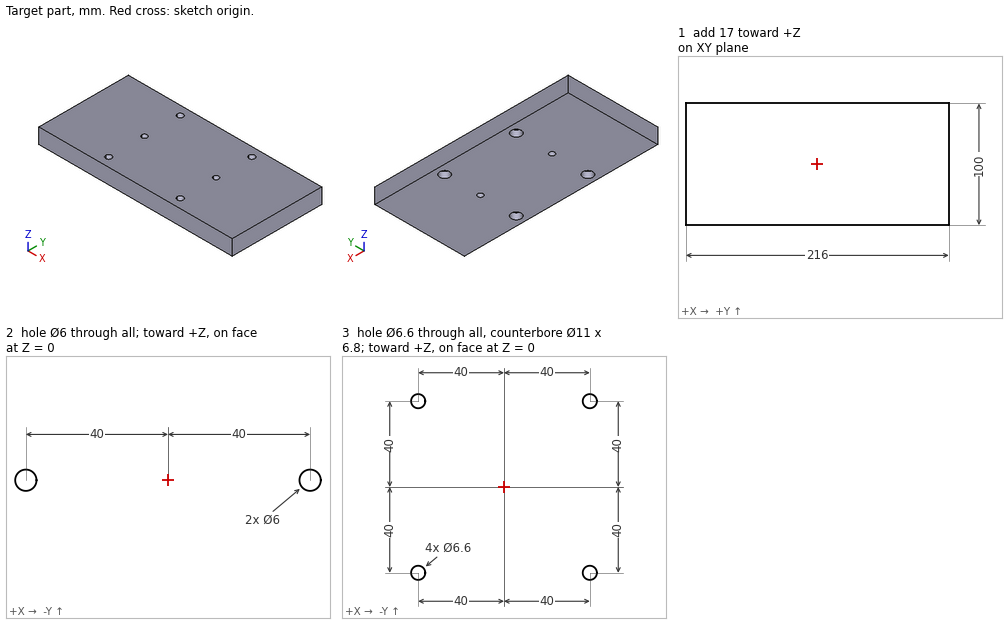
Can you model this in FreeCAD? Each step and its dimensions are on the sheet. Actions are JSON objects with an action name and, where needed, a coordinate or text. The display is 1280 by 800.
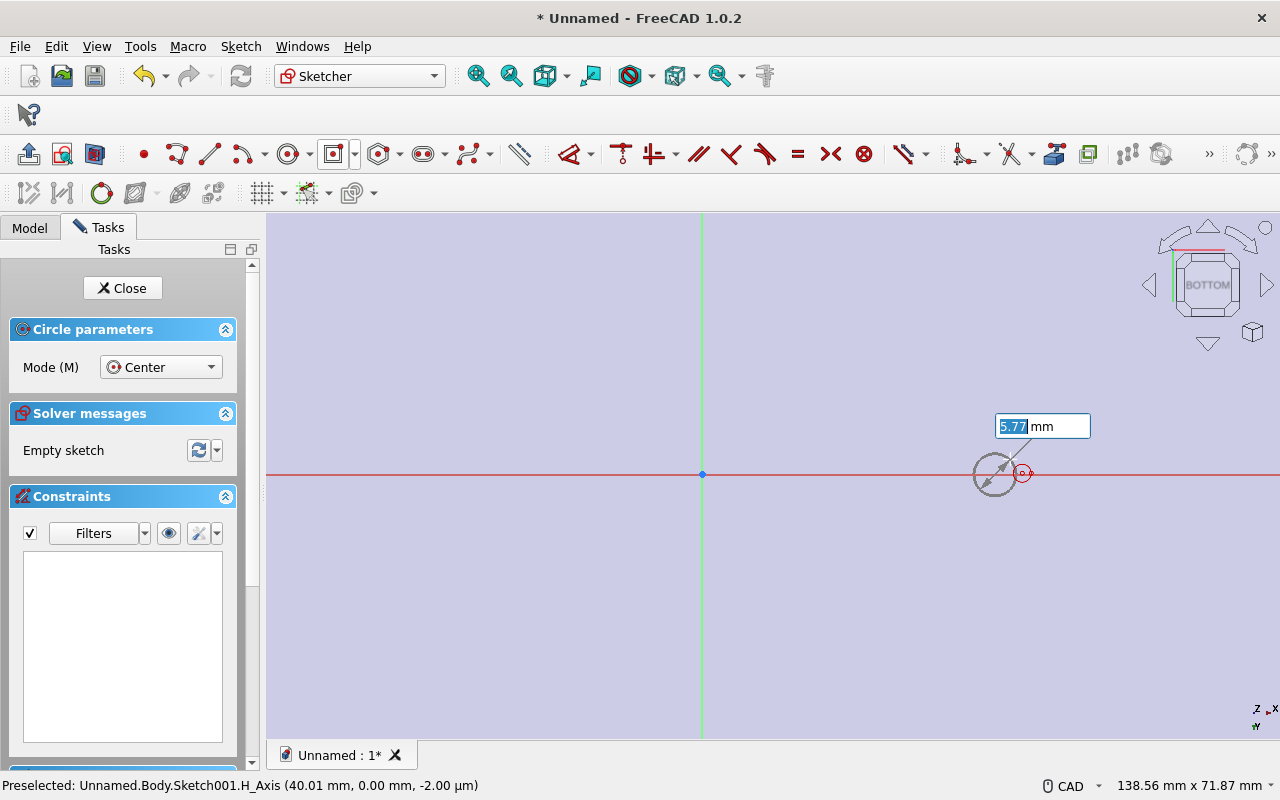
{"action": "type", "text": "6"}
{"action": "key", "text": "Return"}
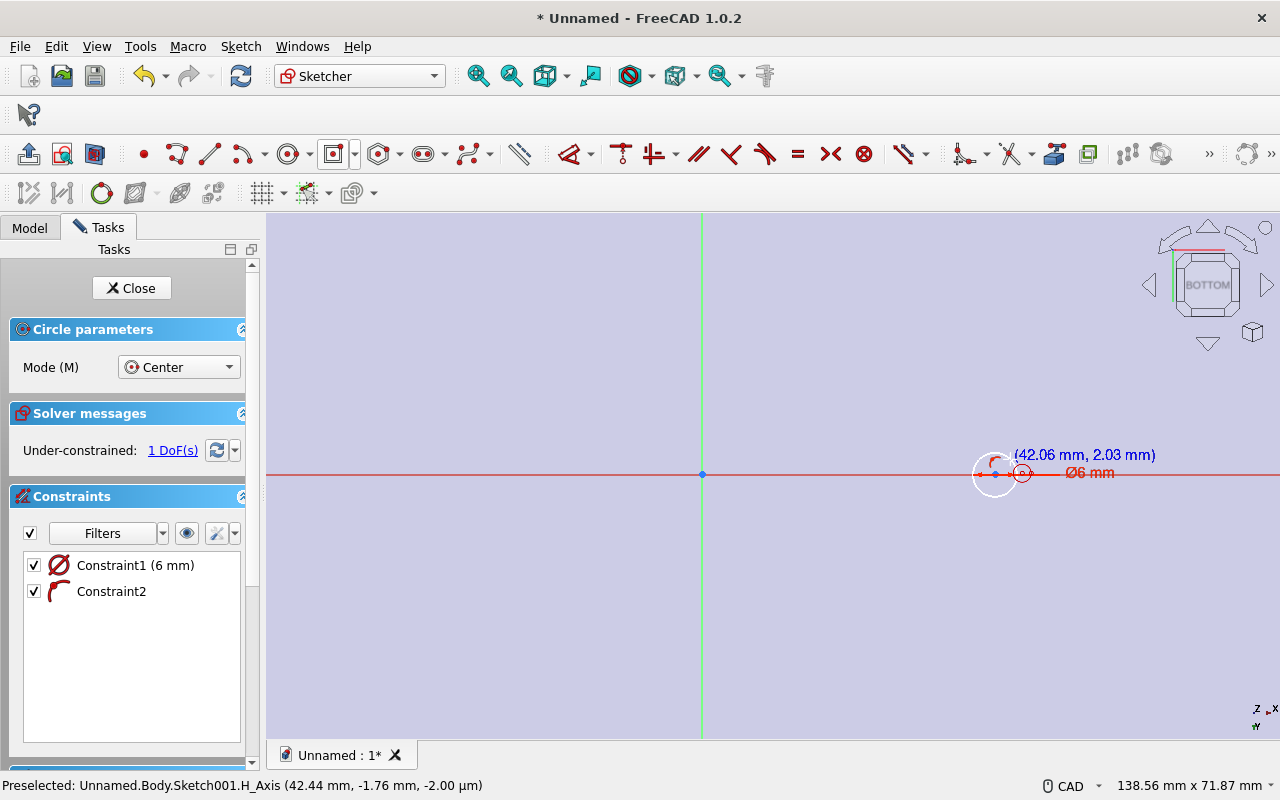
{"action": "left_click", "coordinate": [409, 475]}
{"action": "mouse_move", "coordinate": [425, 459]}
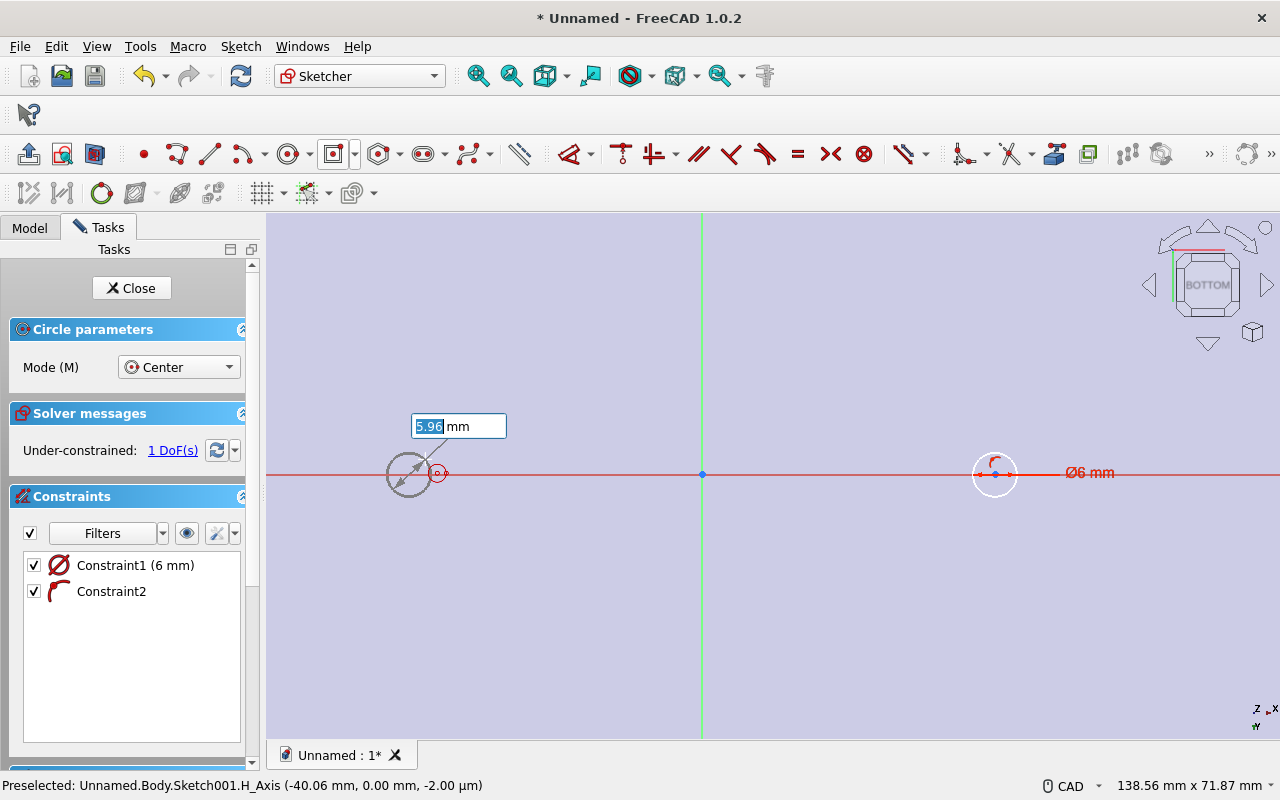
{"action": "type", "text": "6"}
{"action": "key", "text": "Return"}
{"action": "key", "text": "Escape"}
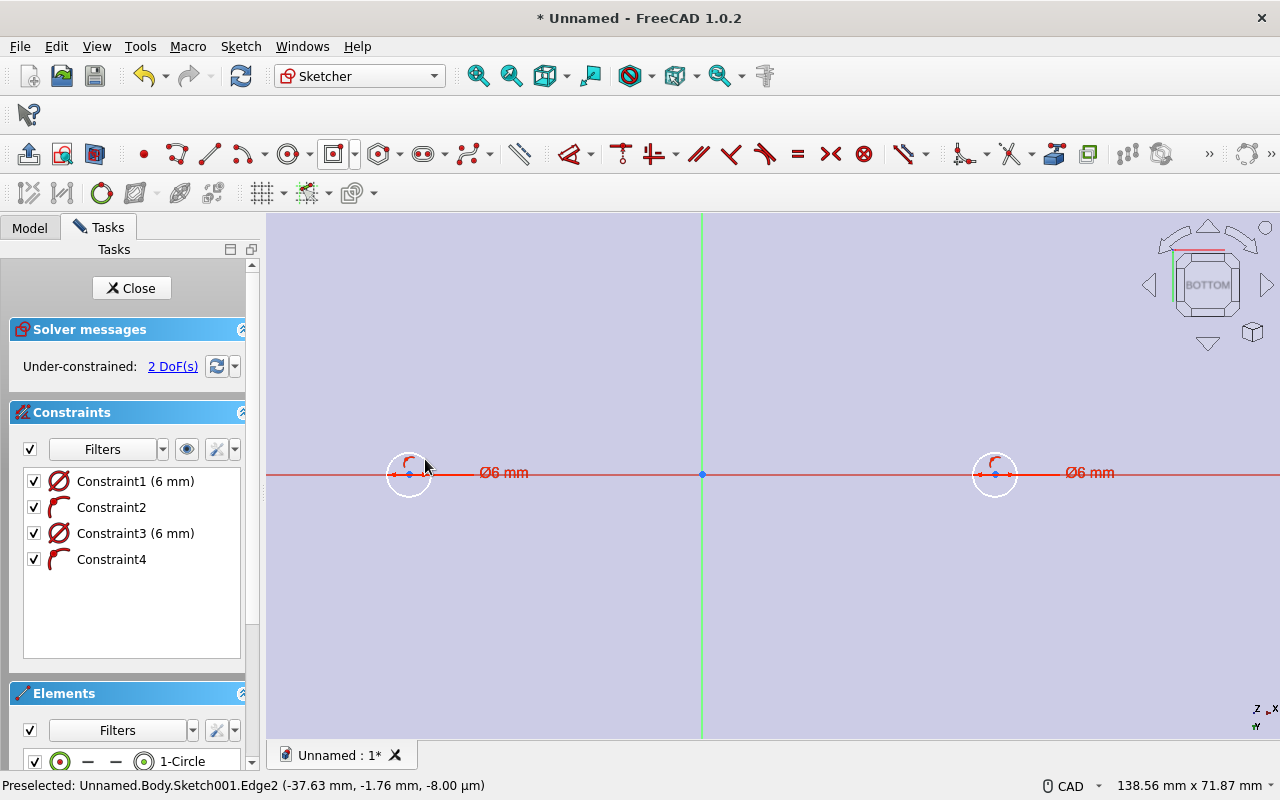
{"action": "left_click", "coordinate": [568, 154]}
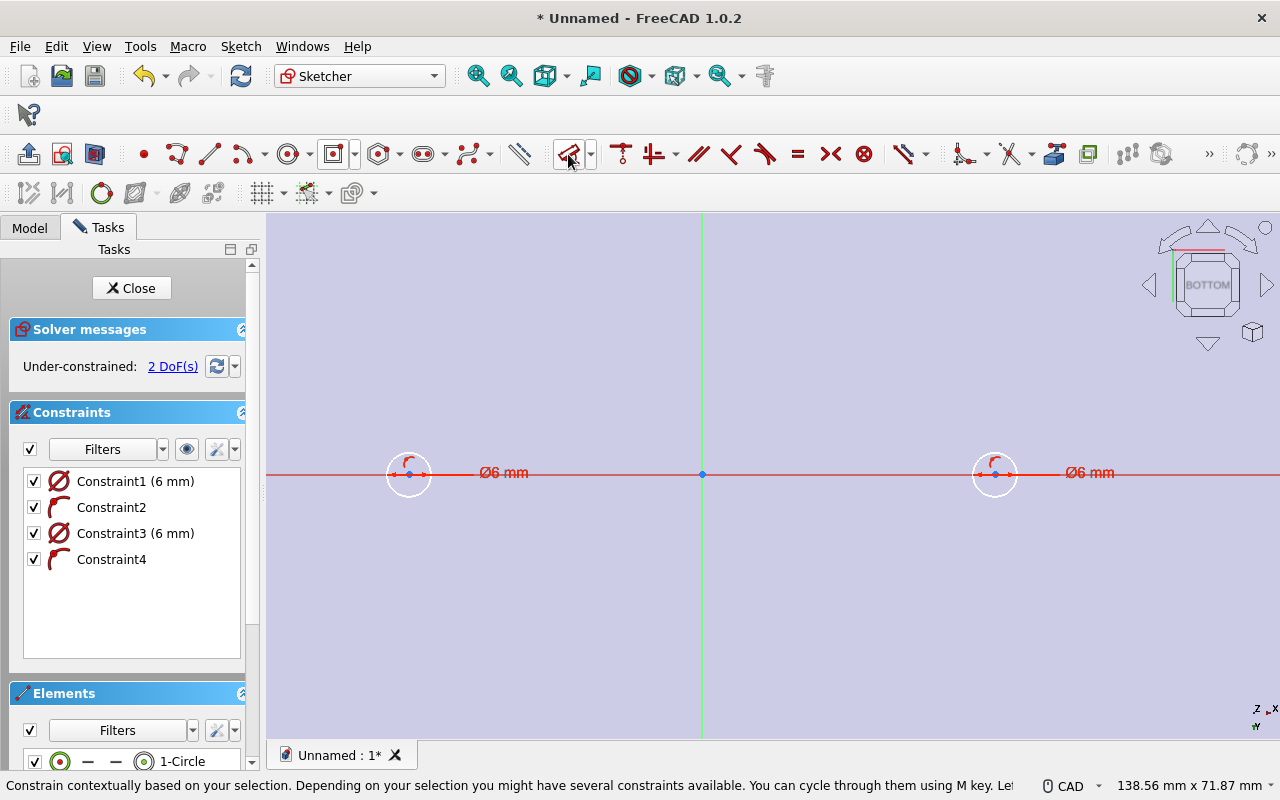
{"action": "left_click", "coordinate": [995, 475]}
{"action": "left_click", "coordinate": [849, 509]}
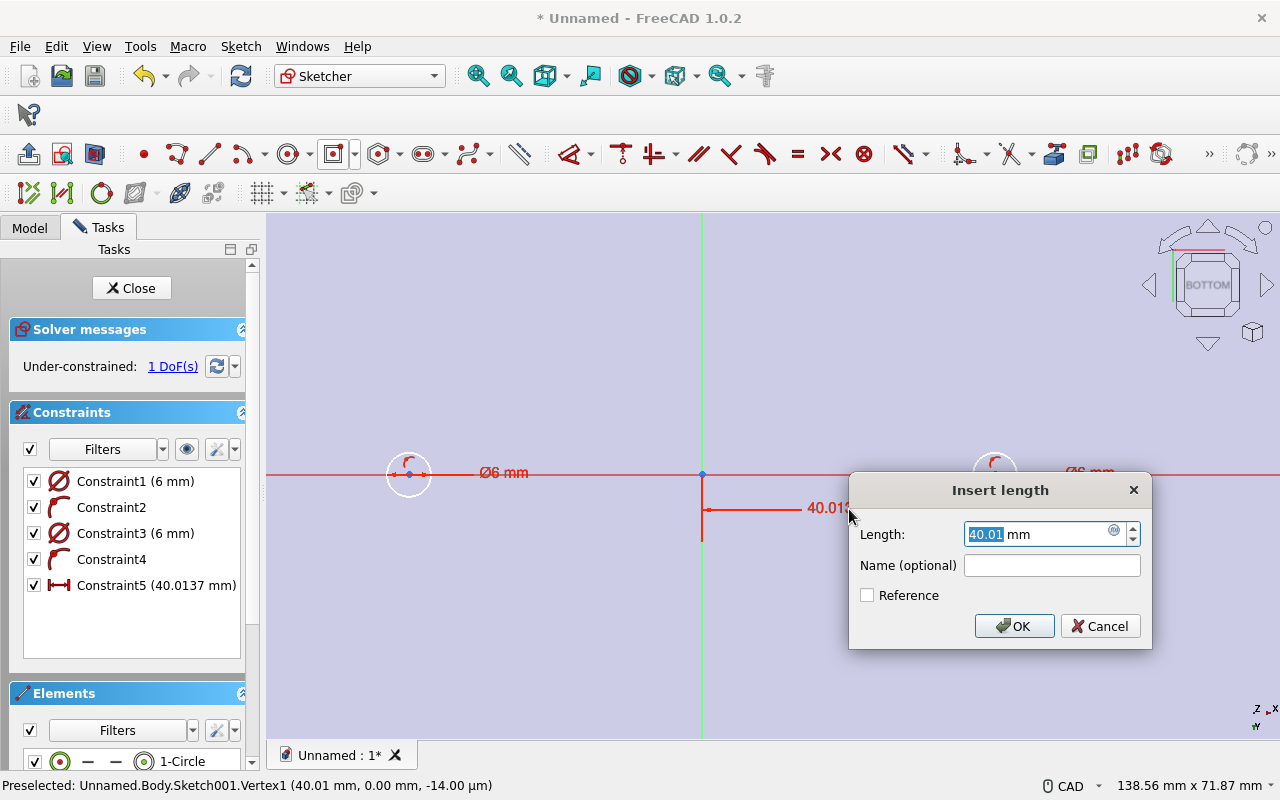
{"action": "type", "text": "40"}
{"action": "key", "text": "Return"}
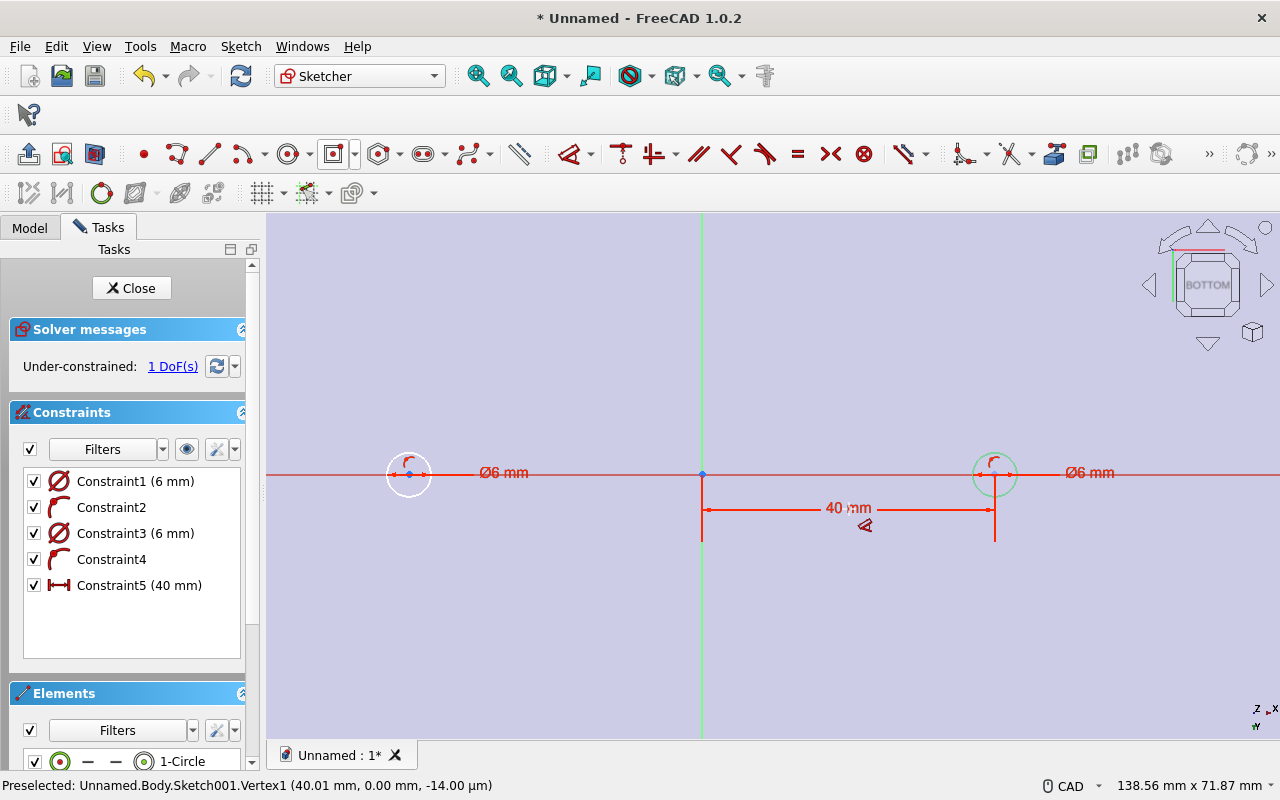
{"action": "left_click", "coordinate": [409, 475]}
{"action": "left_click", "coordinate": [556, 509]}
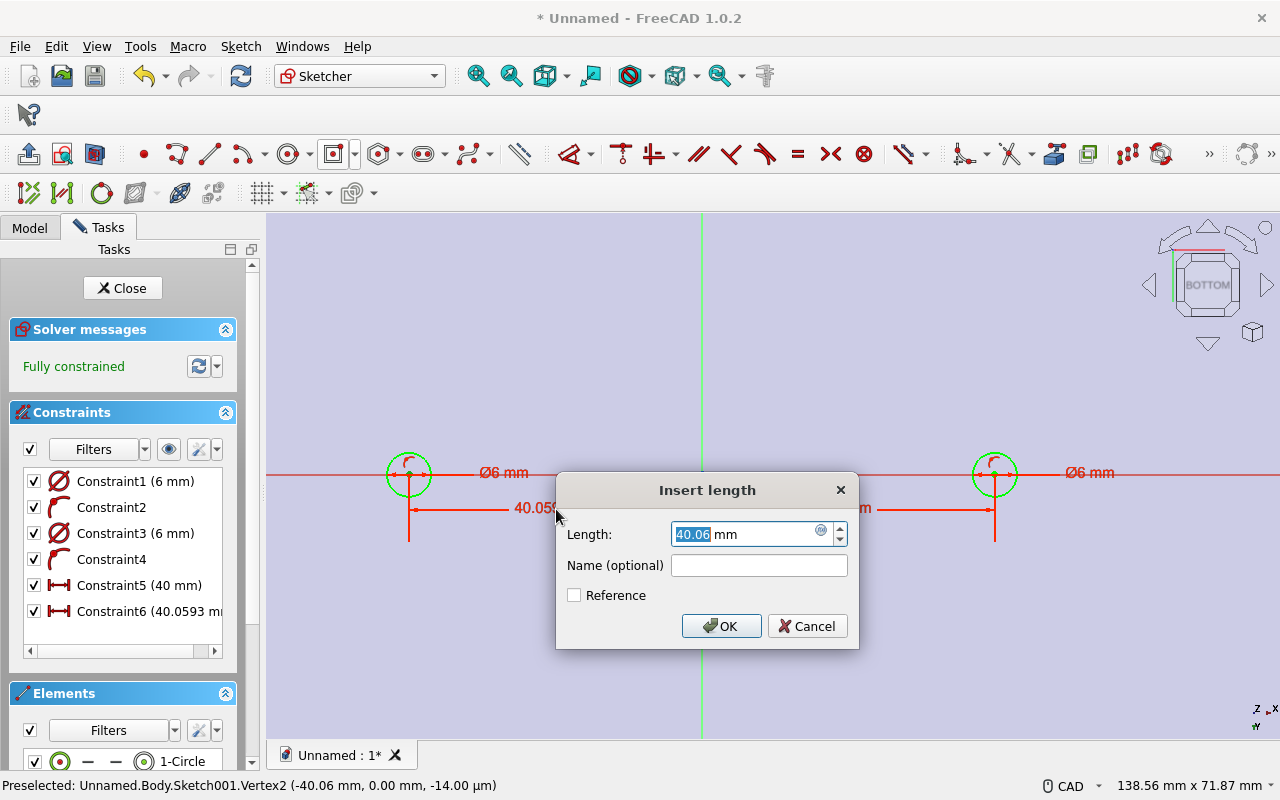
{"action": "type", "text": "40"}
{"action": "key", "text": "Return"}
{"action": "key", "text": "Escape"}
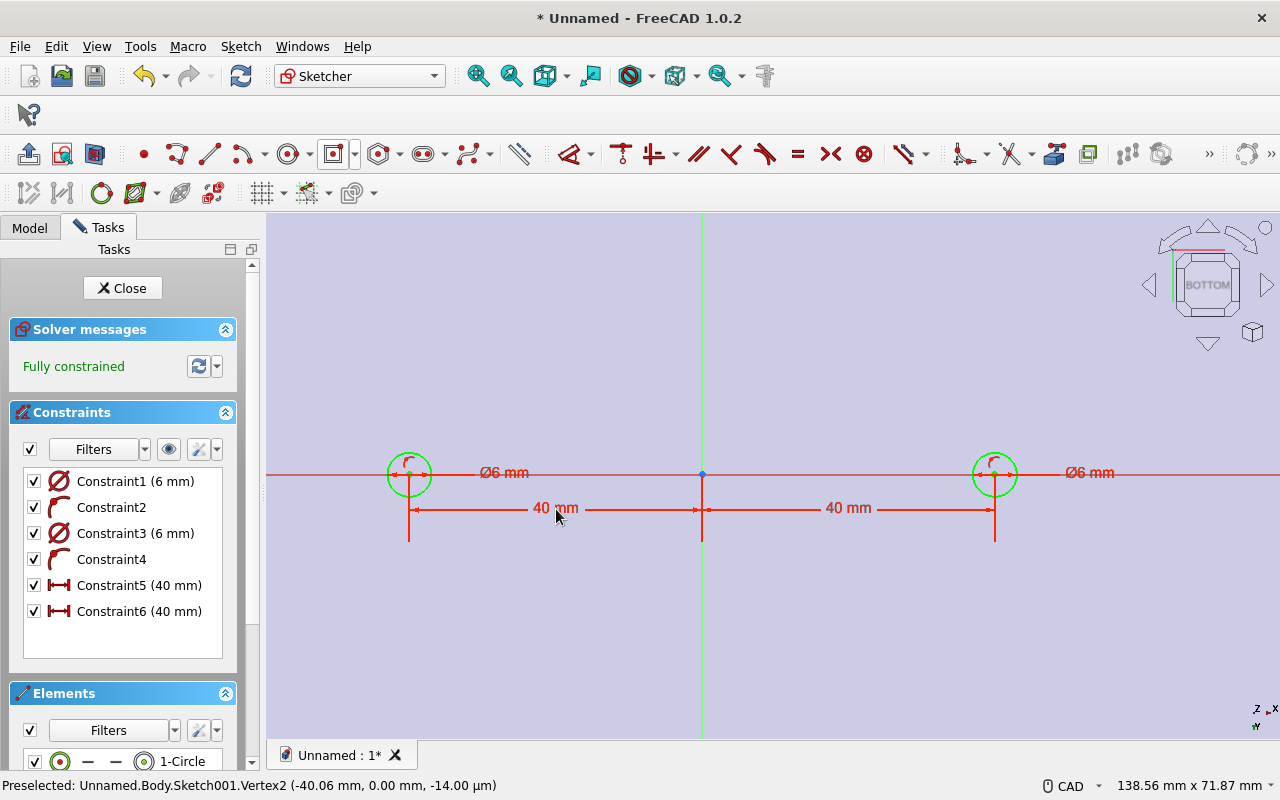
{"action": "left_click", "coordinate": [123, 288]}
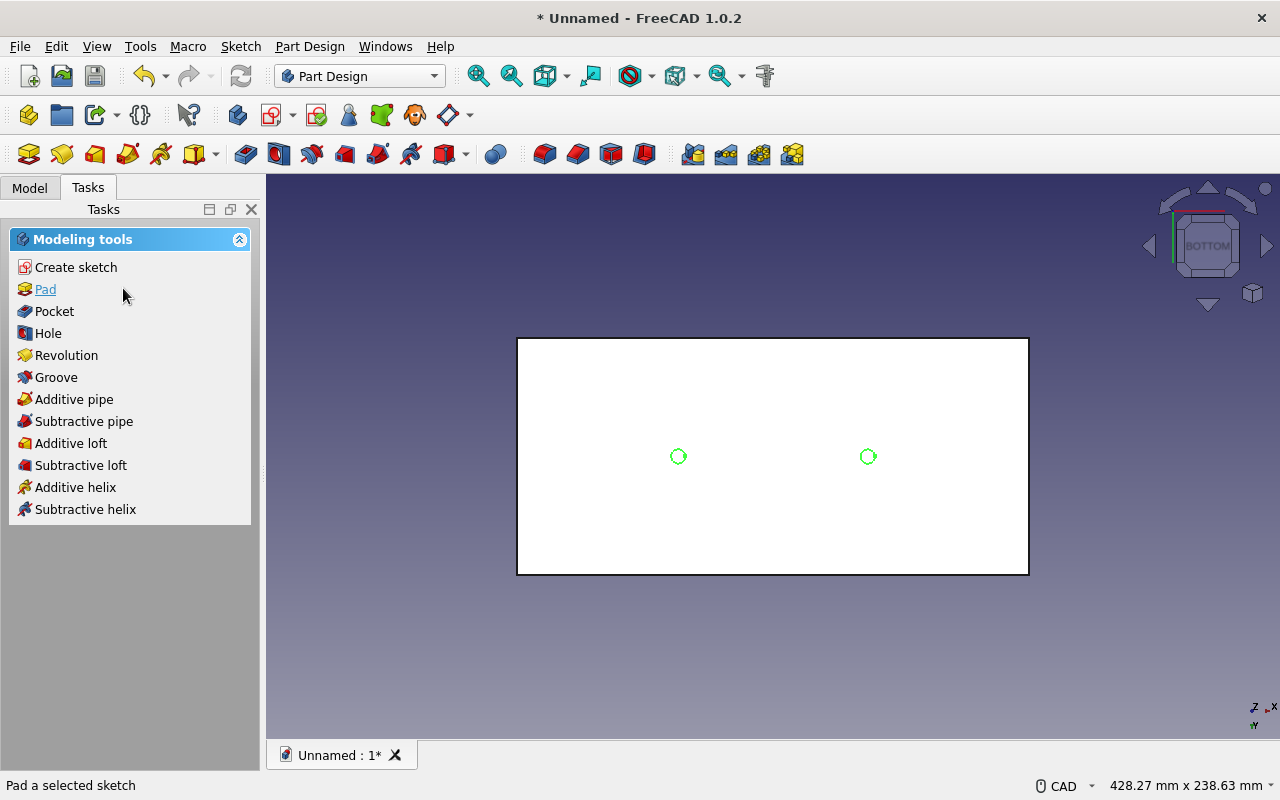
{"action": "left_click", "coordinate": [279, 154]}